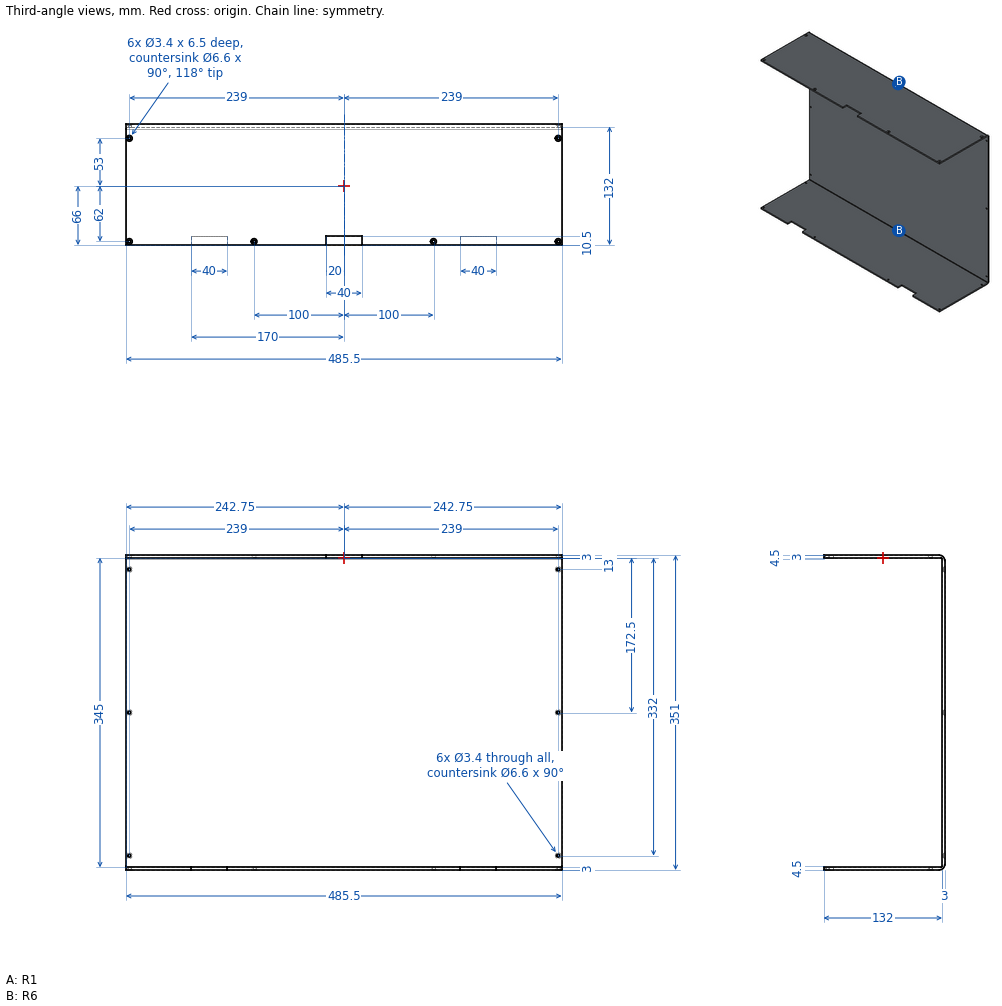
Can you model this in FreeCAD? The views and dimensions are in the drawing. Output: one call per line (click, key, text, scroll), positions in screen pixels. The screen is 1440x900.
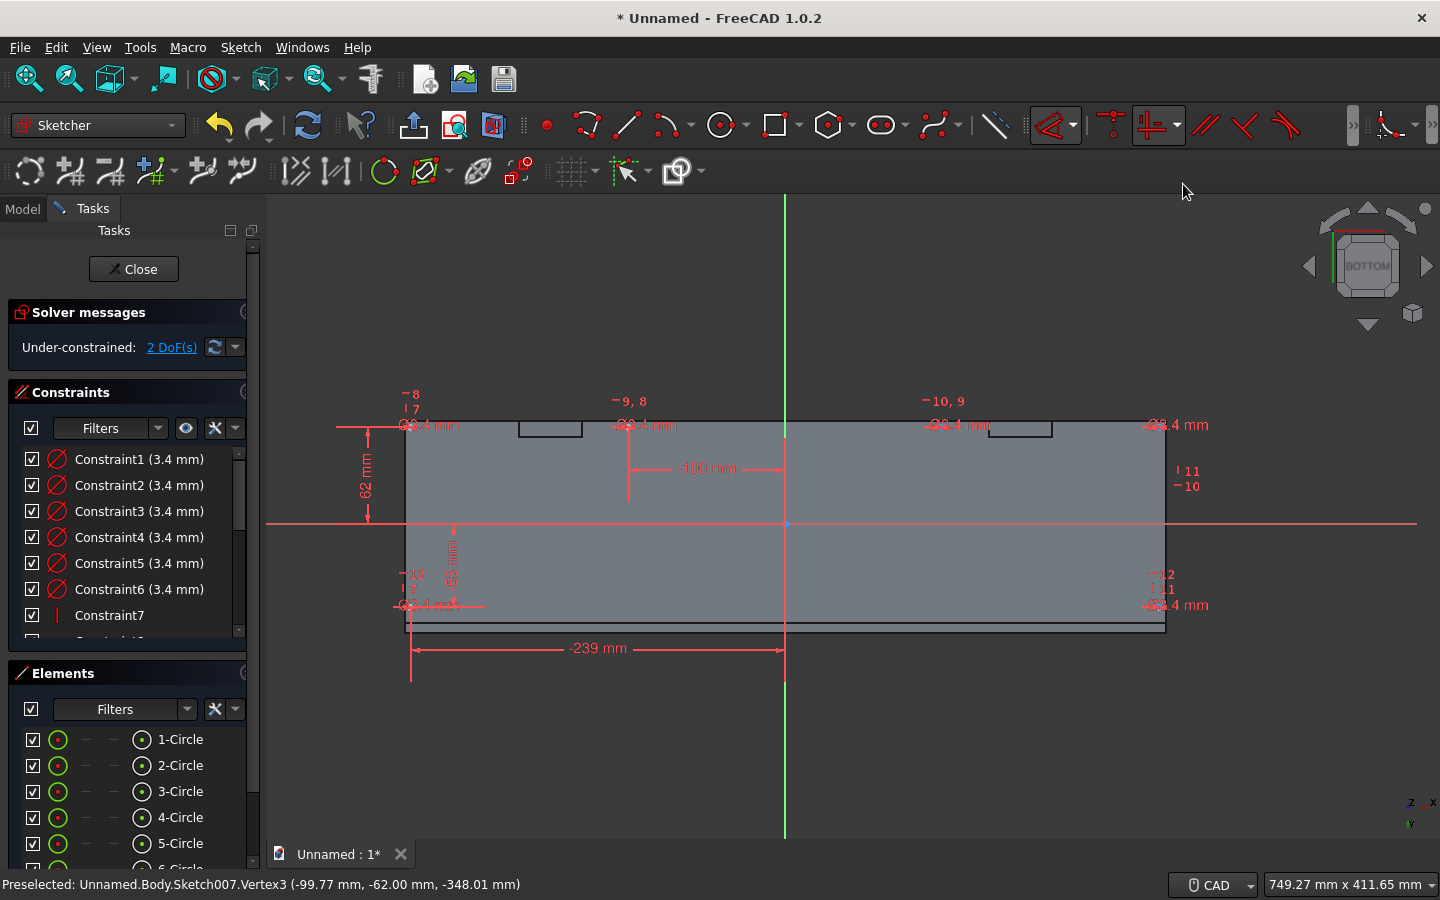
click(942, 427)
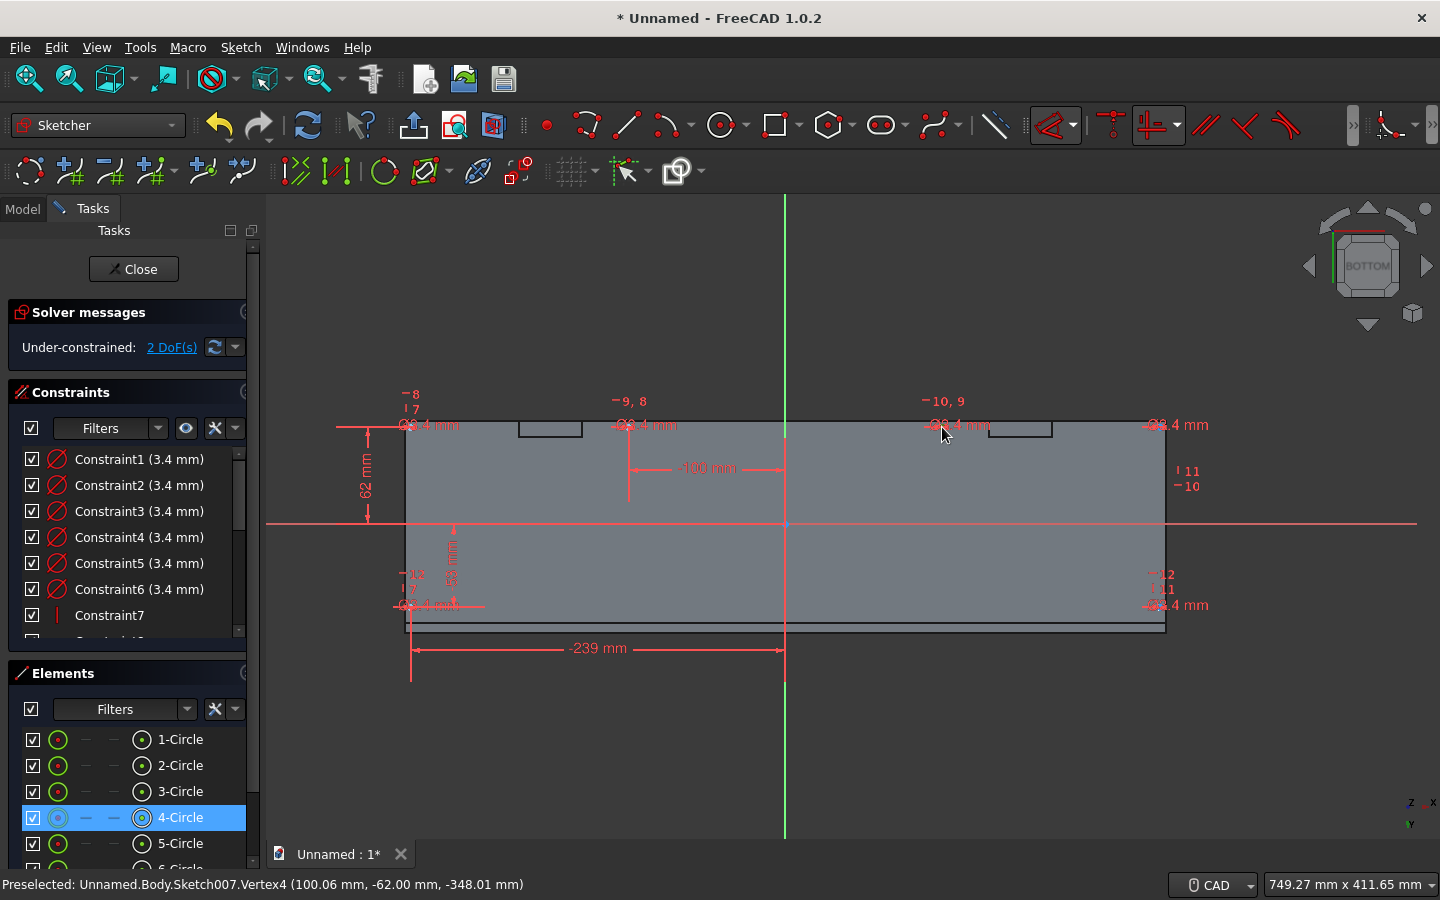
click(1076, 126)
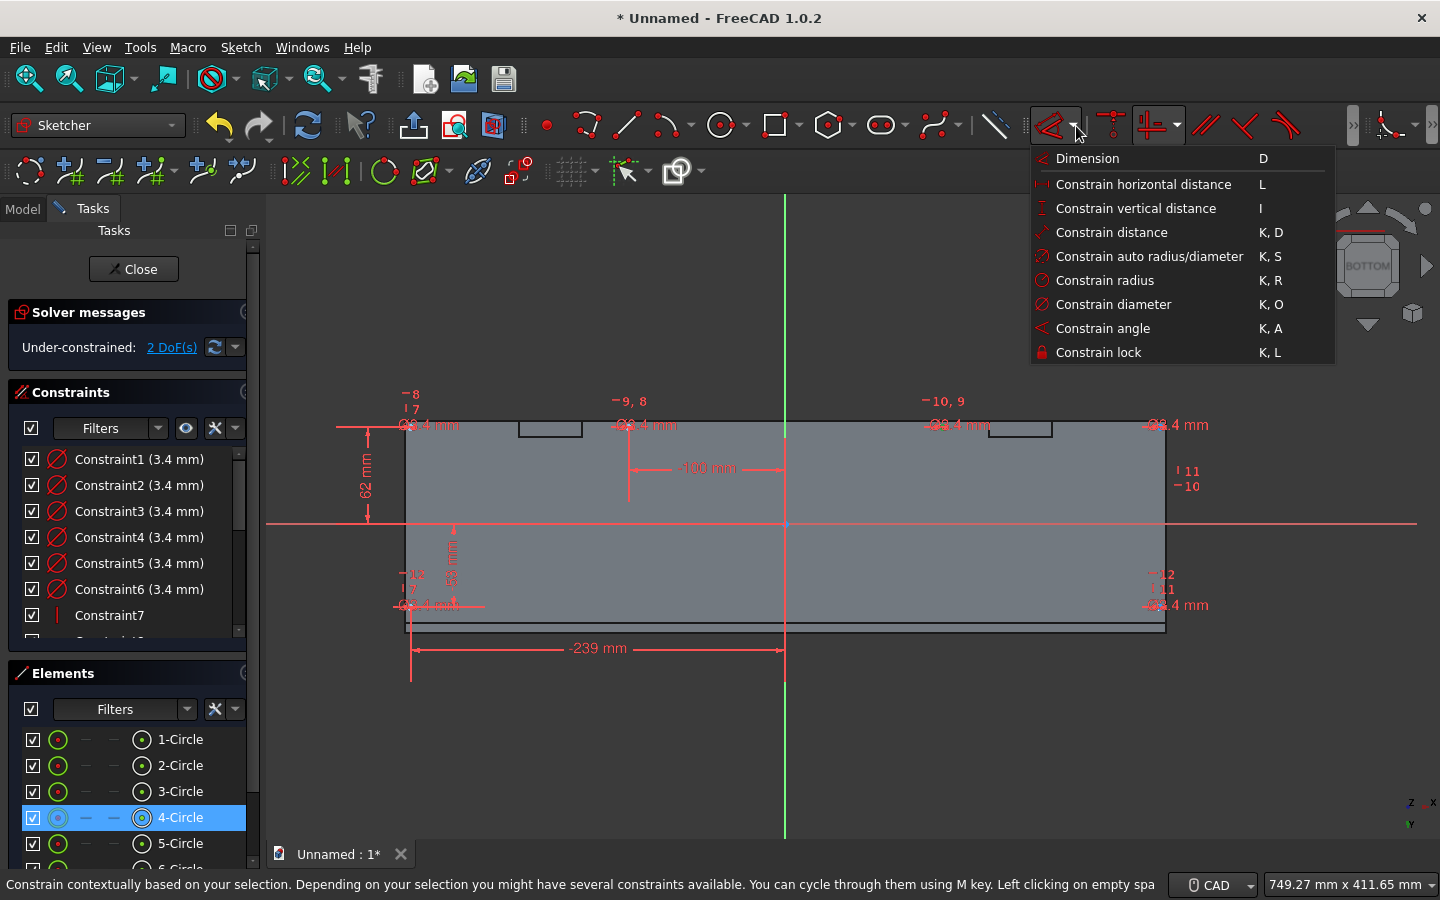
click(1183, 184)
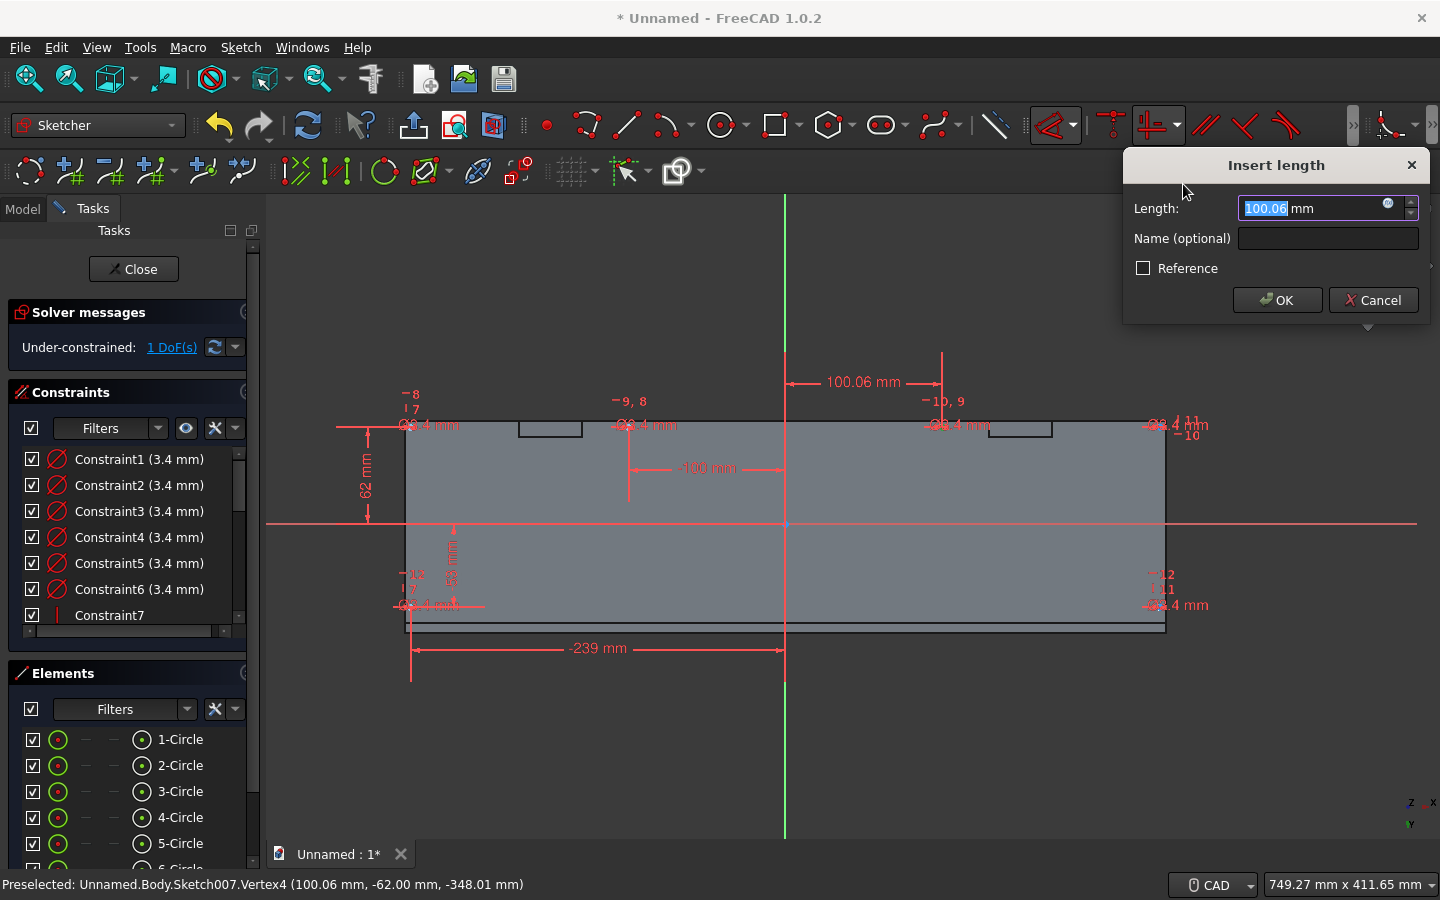
text(100)
key(Return)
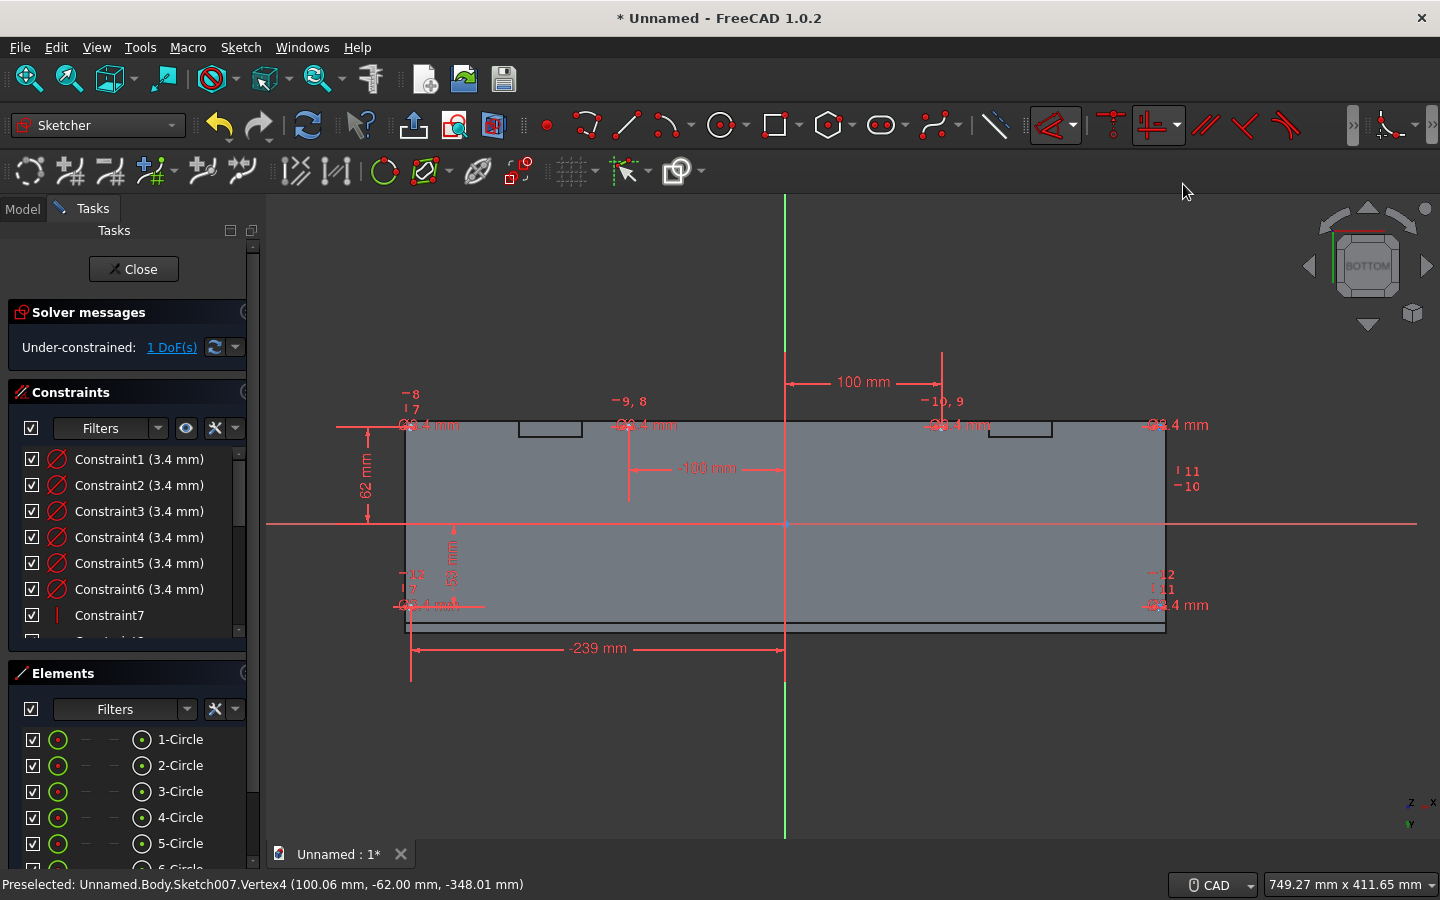
click(1160, 427)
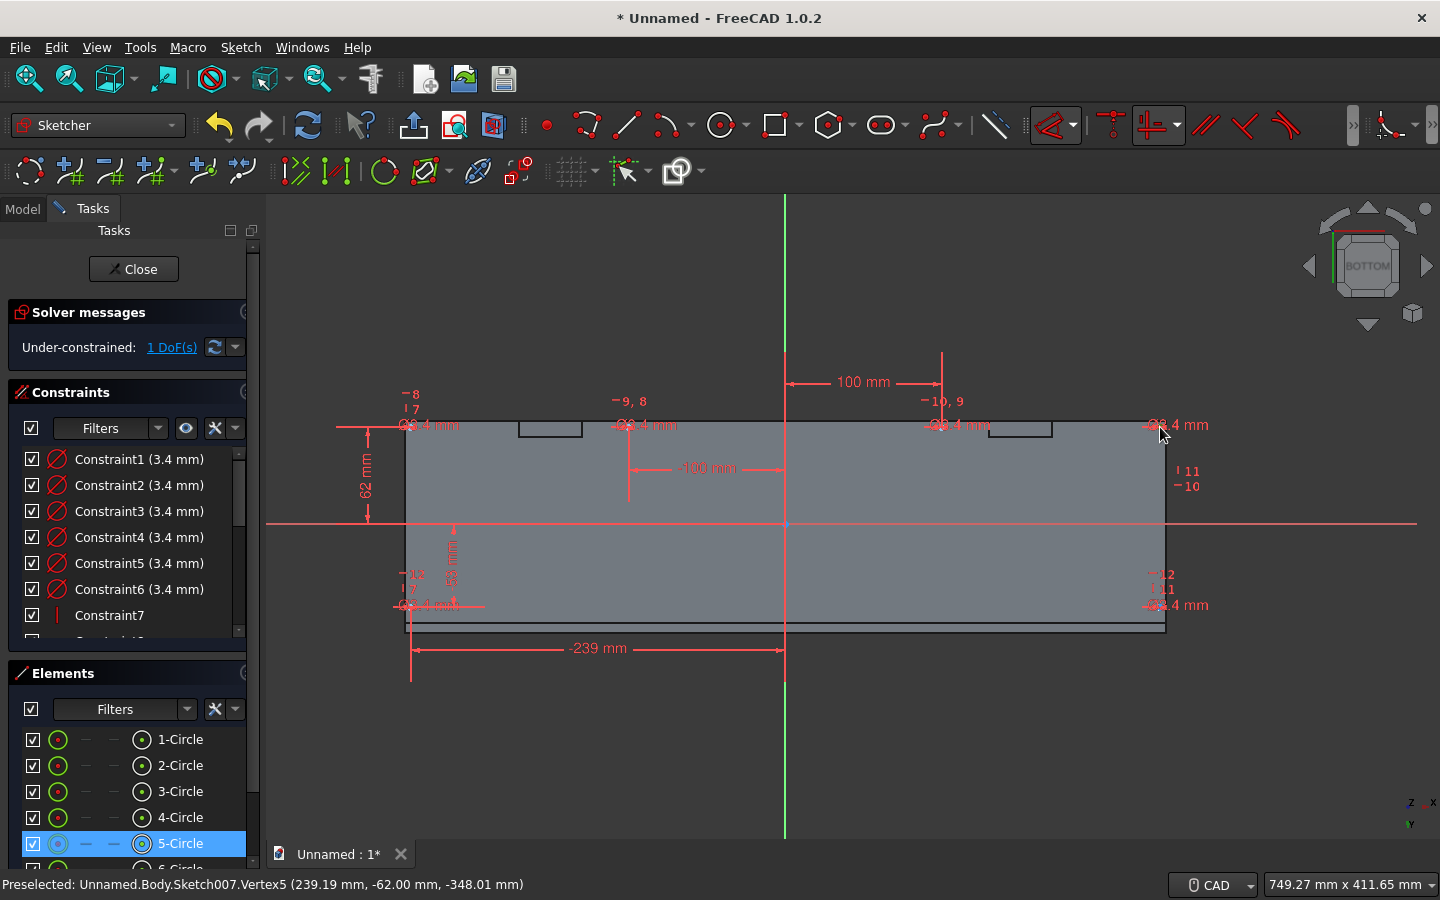
click(1076, 126)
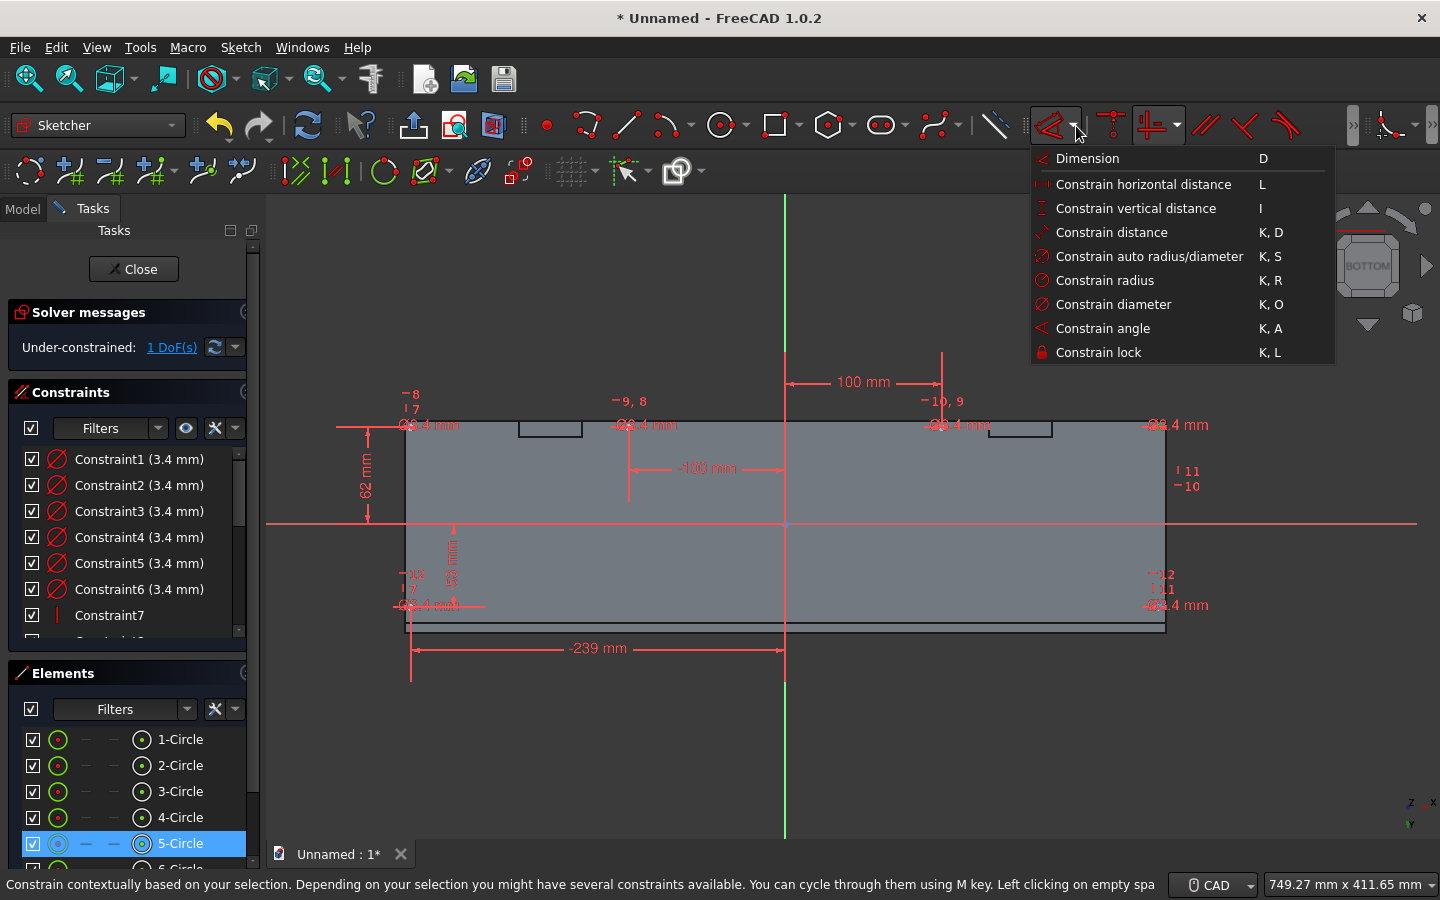
click(1183, 184)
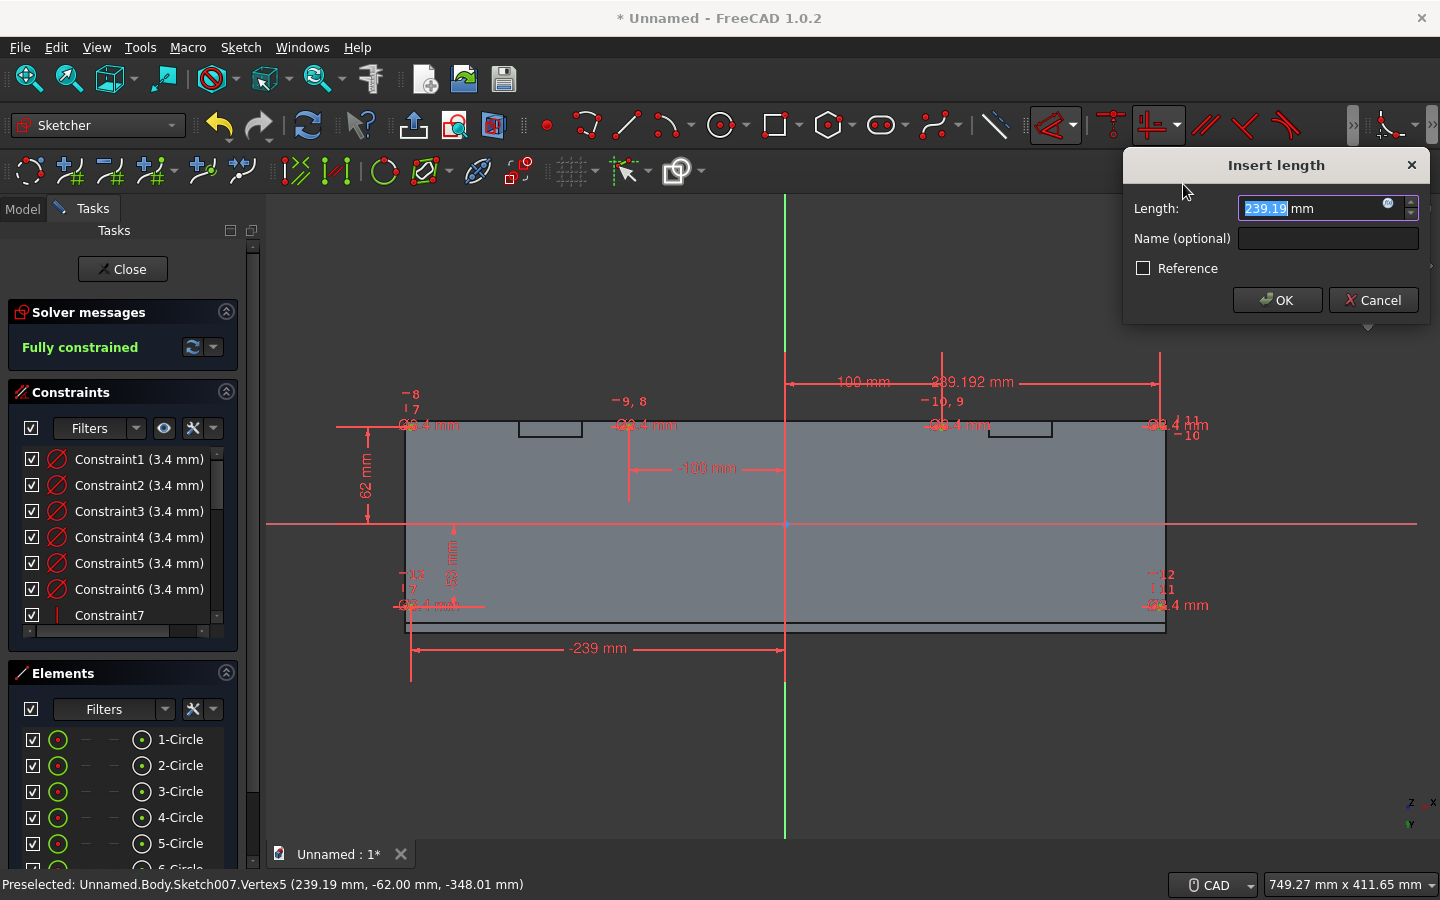
text(239)
key(Return)